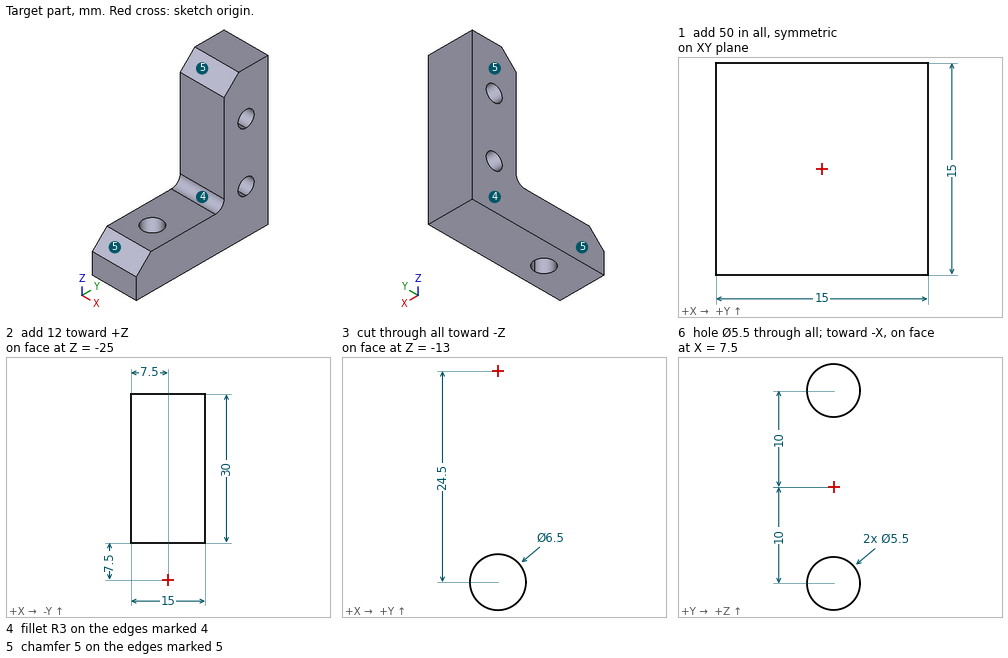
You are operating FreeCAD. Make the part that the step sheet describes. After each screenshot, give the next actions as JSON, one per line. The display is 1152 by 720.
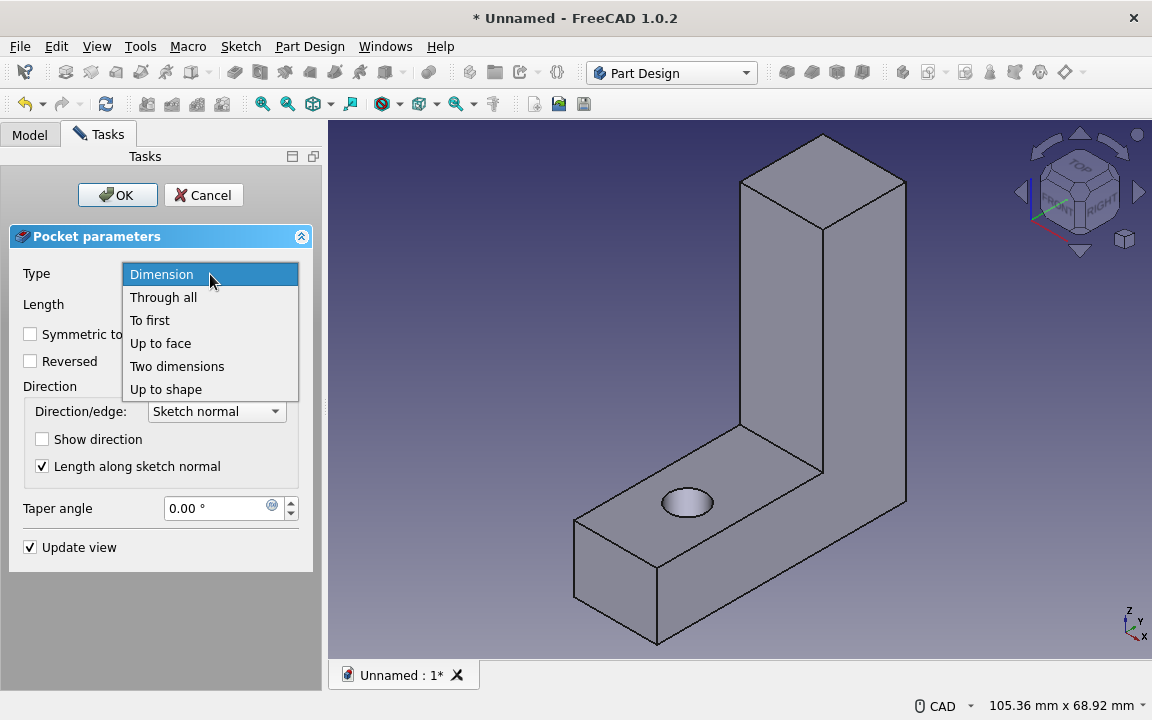
{"action": "left_click", "coordinate": [208, 298]}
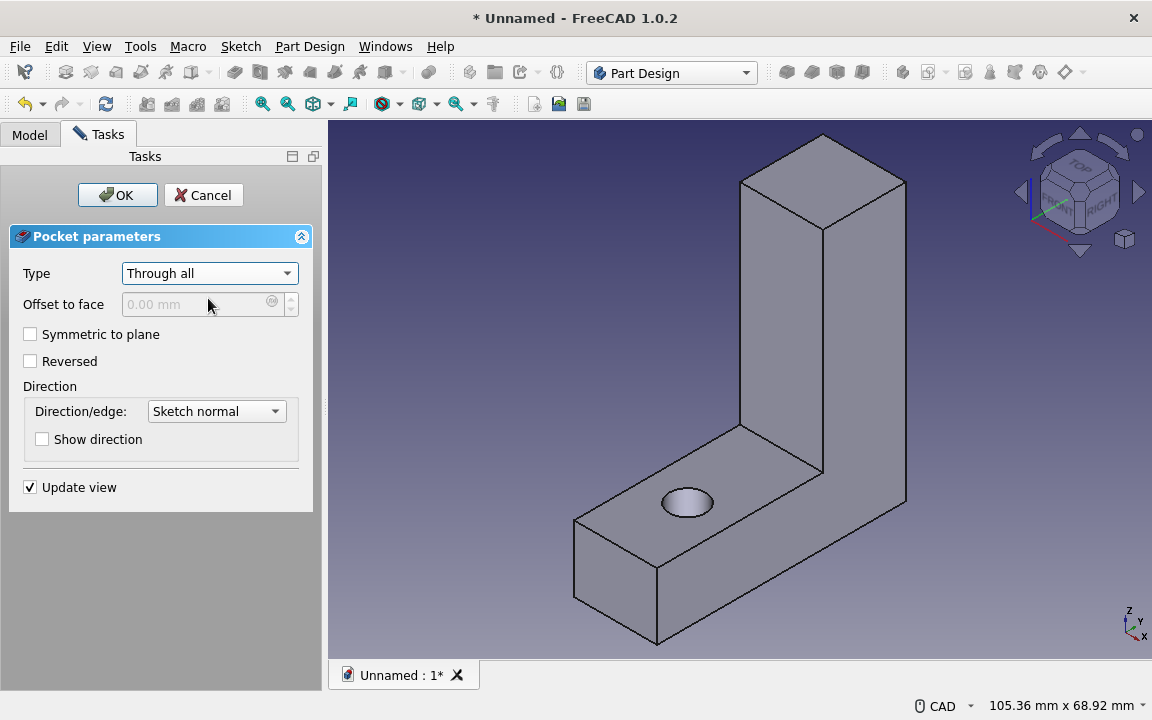
{"action": "left_click", "coordinate": [118, 195]}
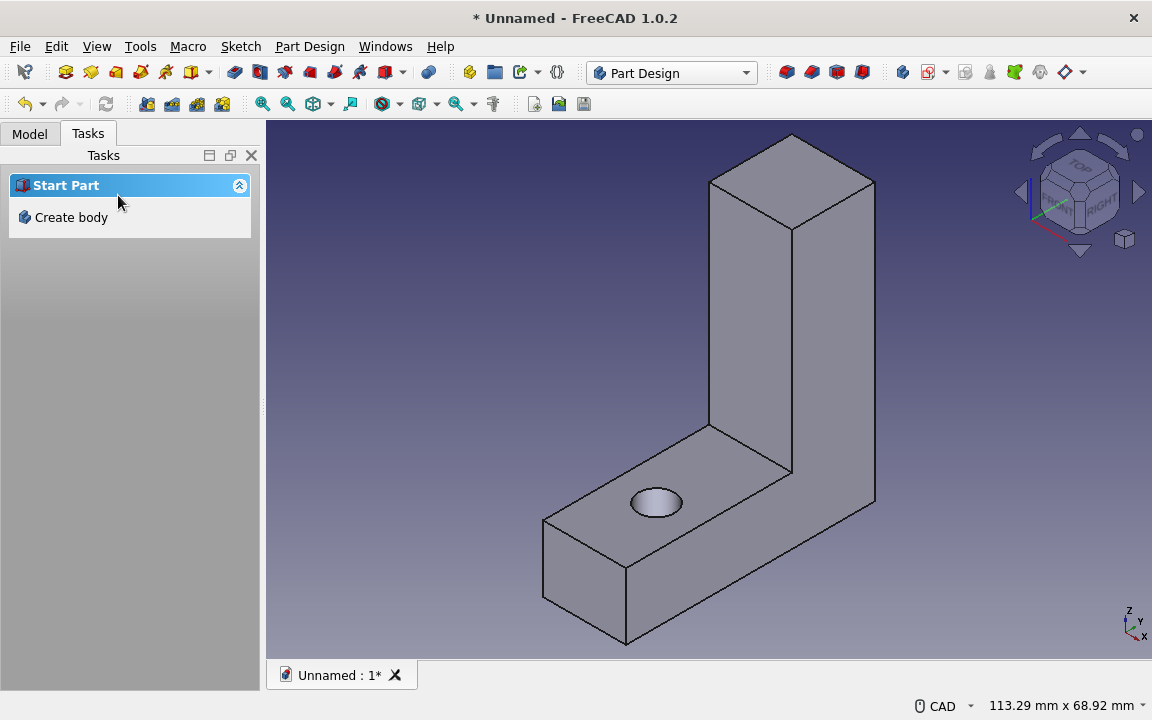
{"action": "key", "text": "2"}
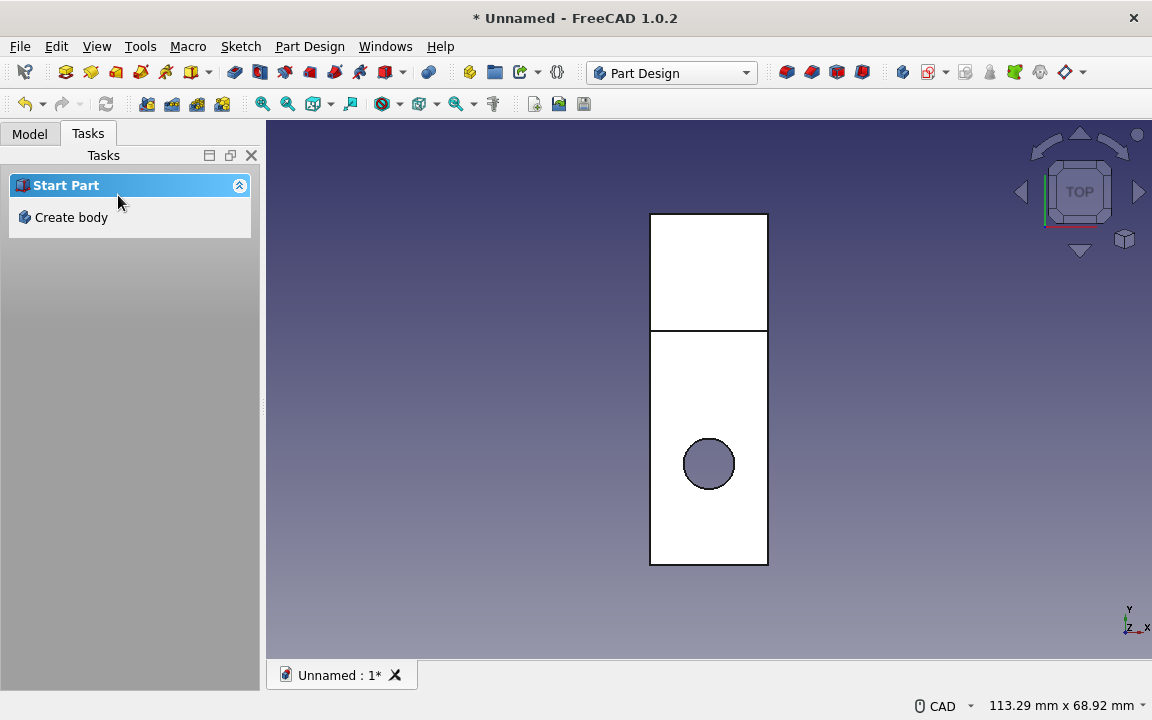
{"action": "key", "text": "0"}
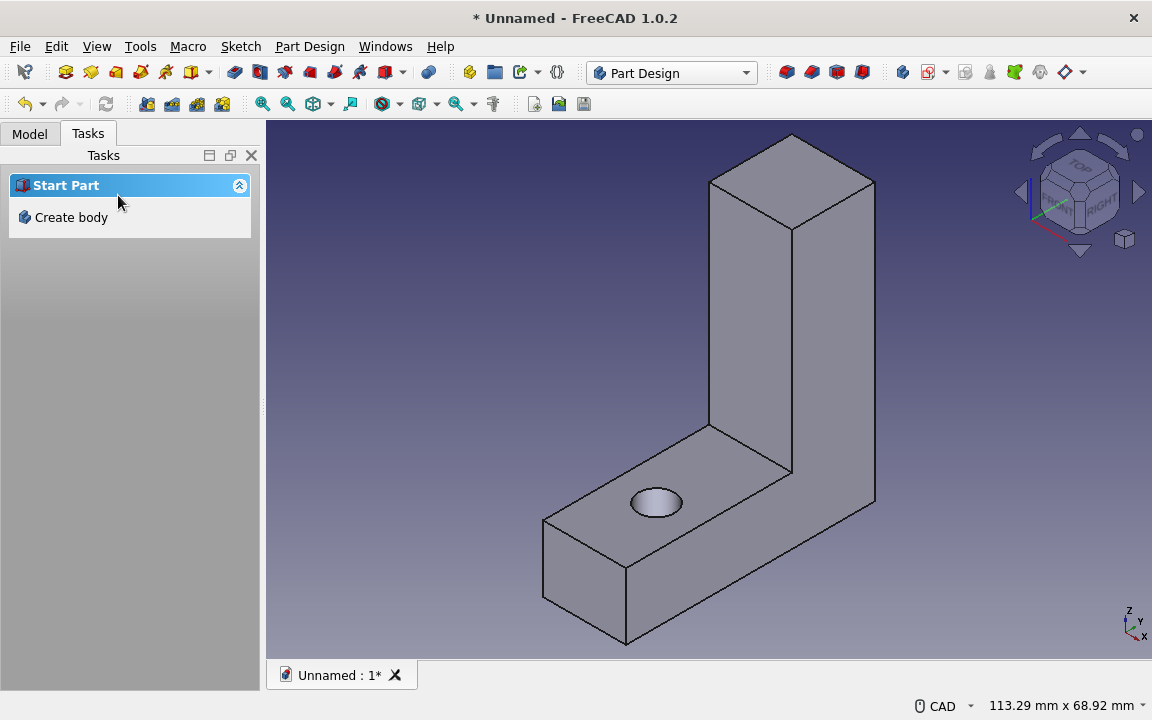
{"action": "key", "text": "1"}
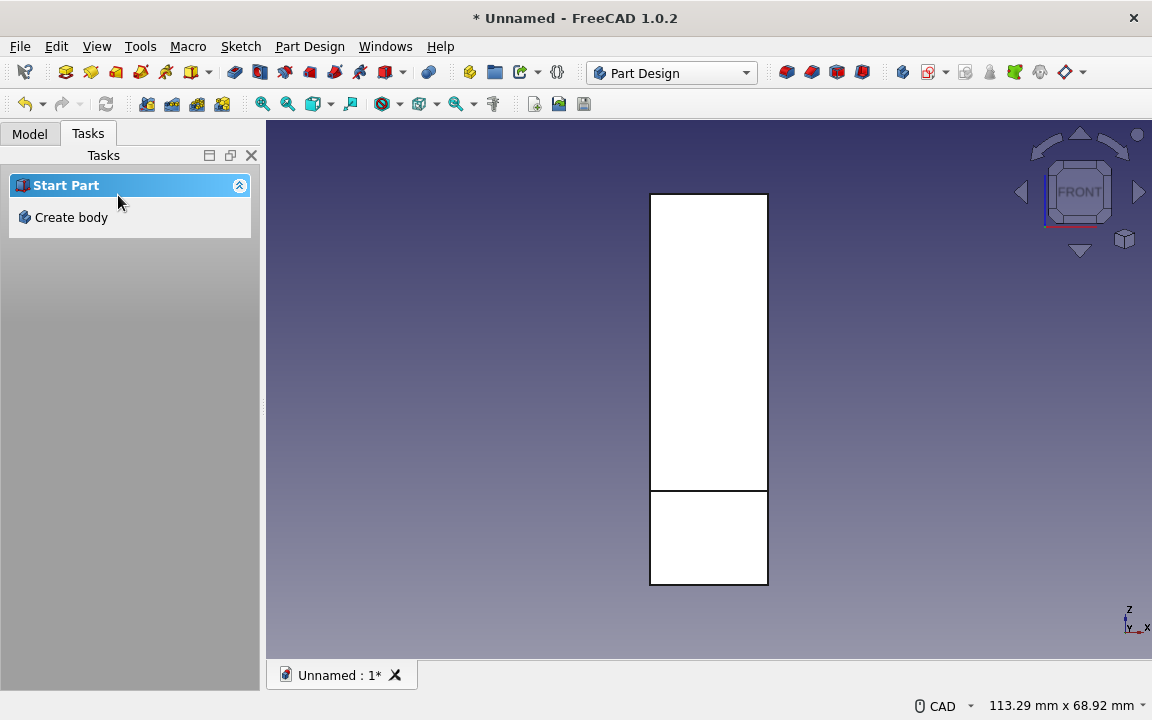
{"action": "key", "text": "3"}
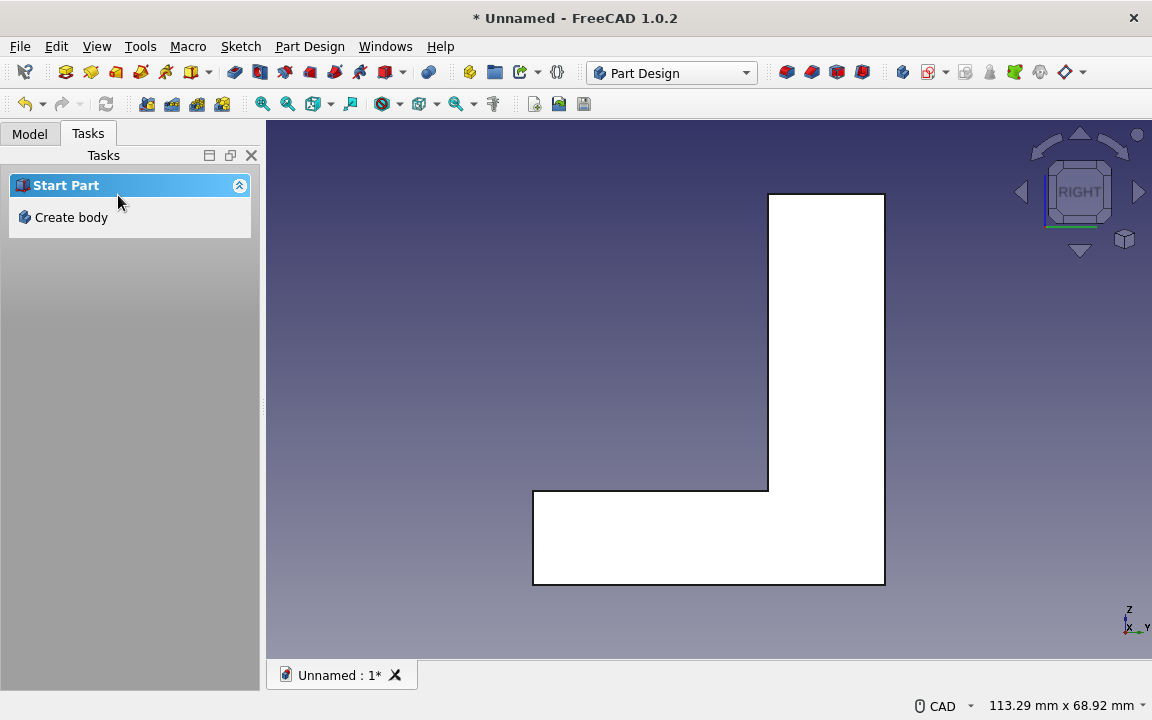
{"action": "key", "text": "5"}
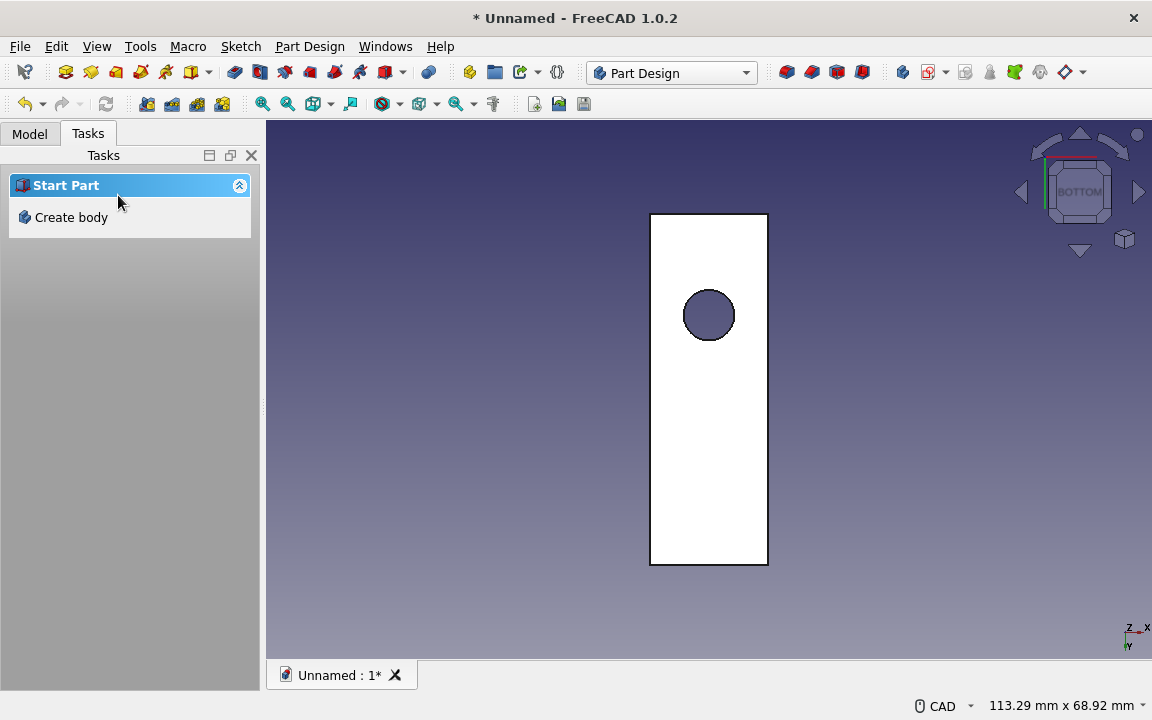
{"action": "key", "text": "4"}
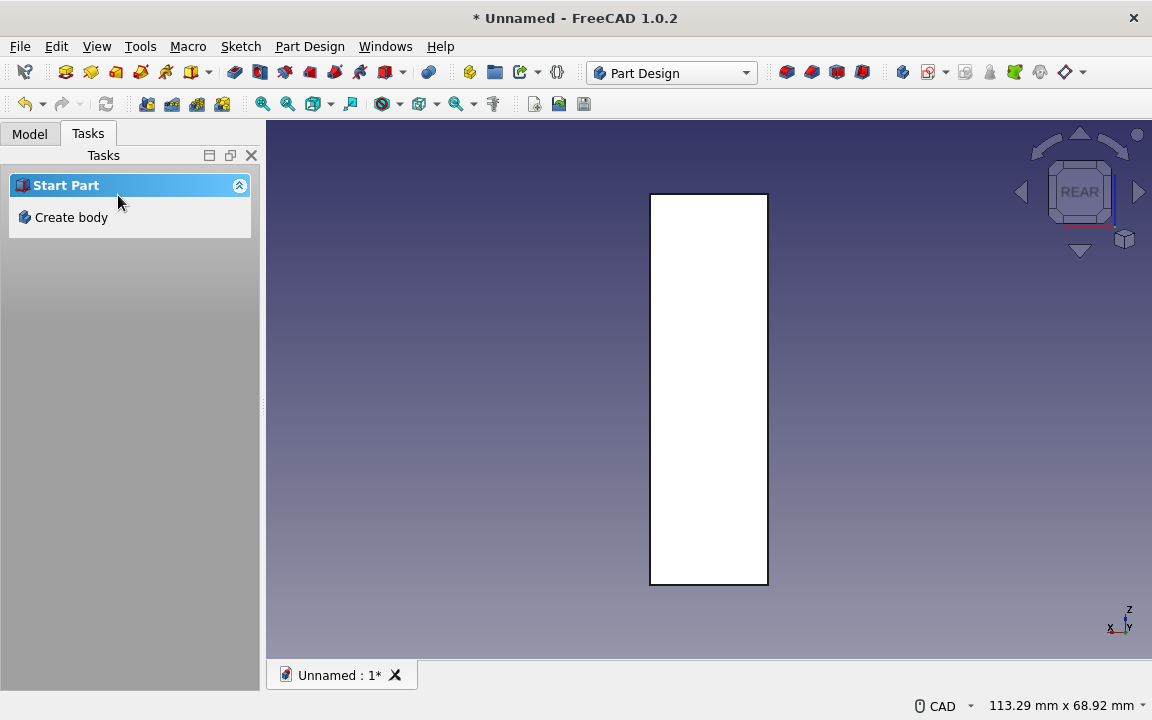
{"action": "key", "text": "6"}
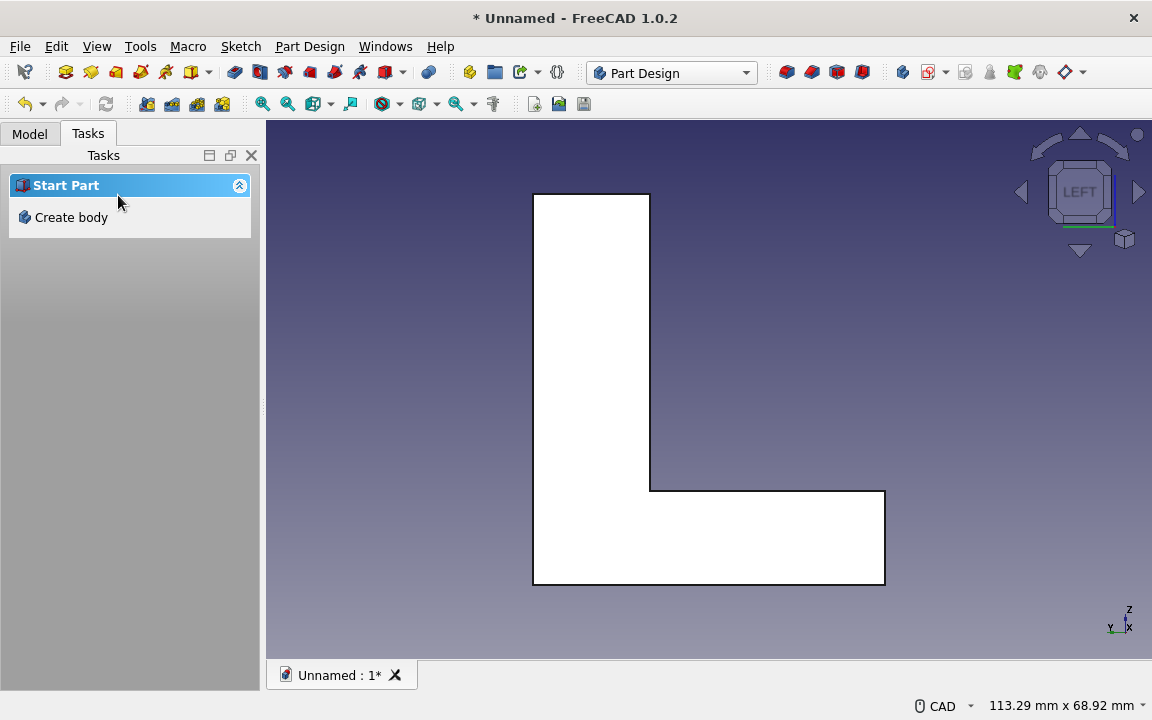
{"action": "key", "text": "v 3"}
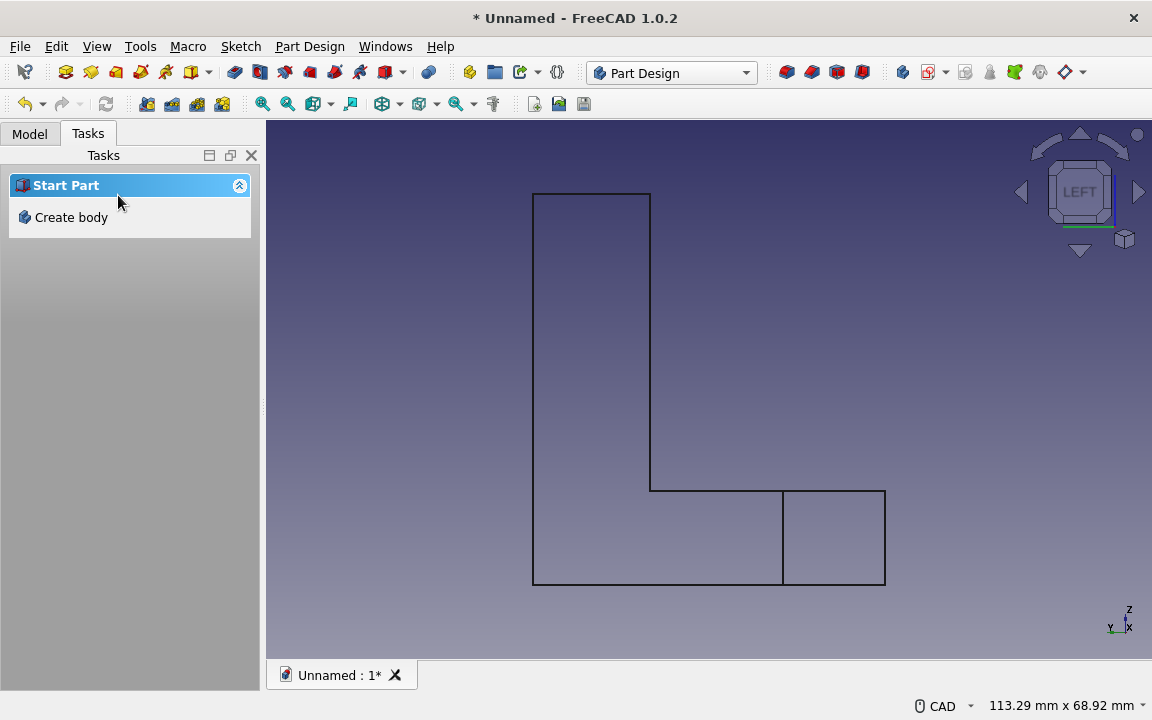
{"action": "key", "text": "0"}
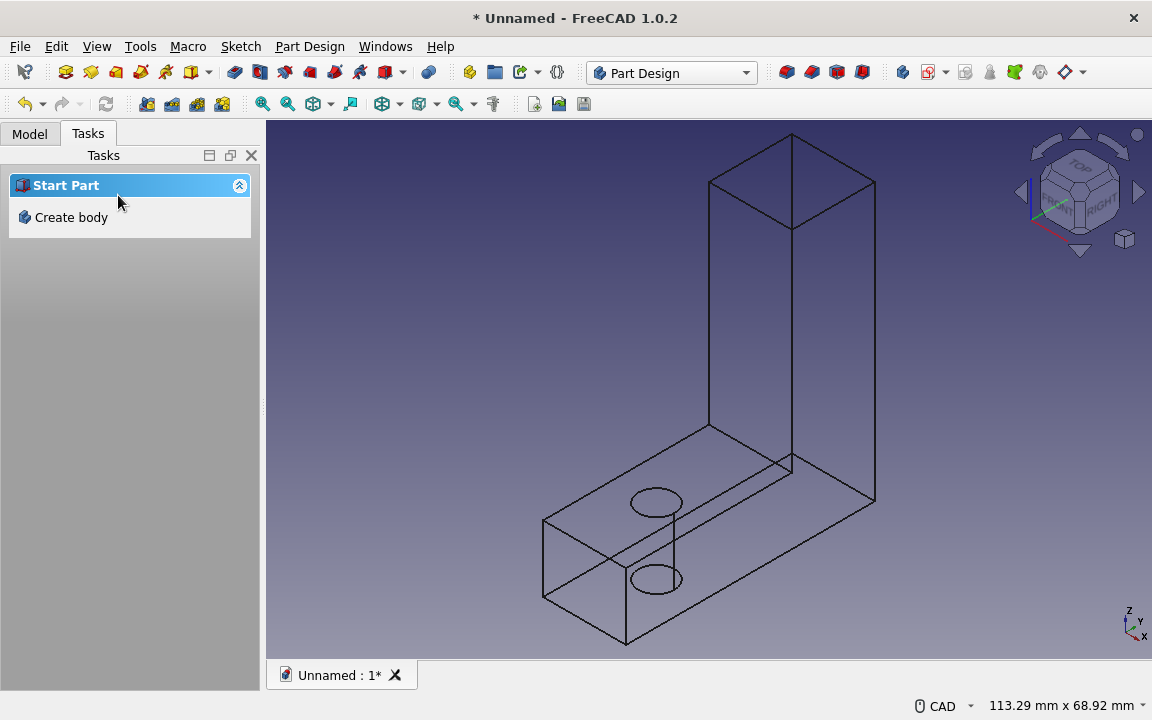
{"action": "left_click", "coordinate": [750, 448]}